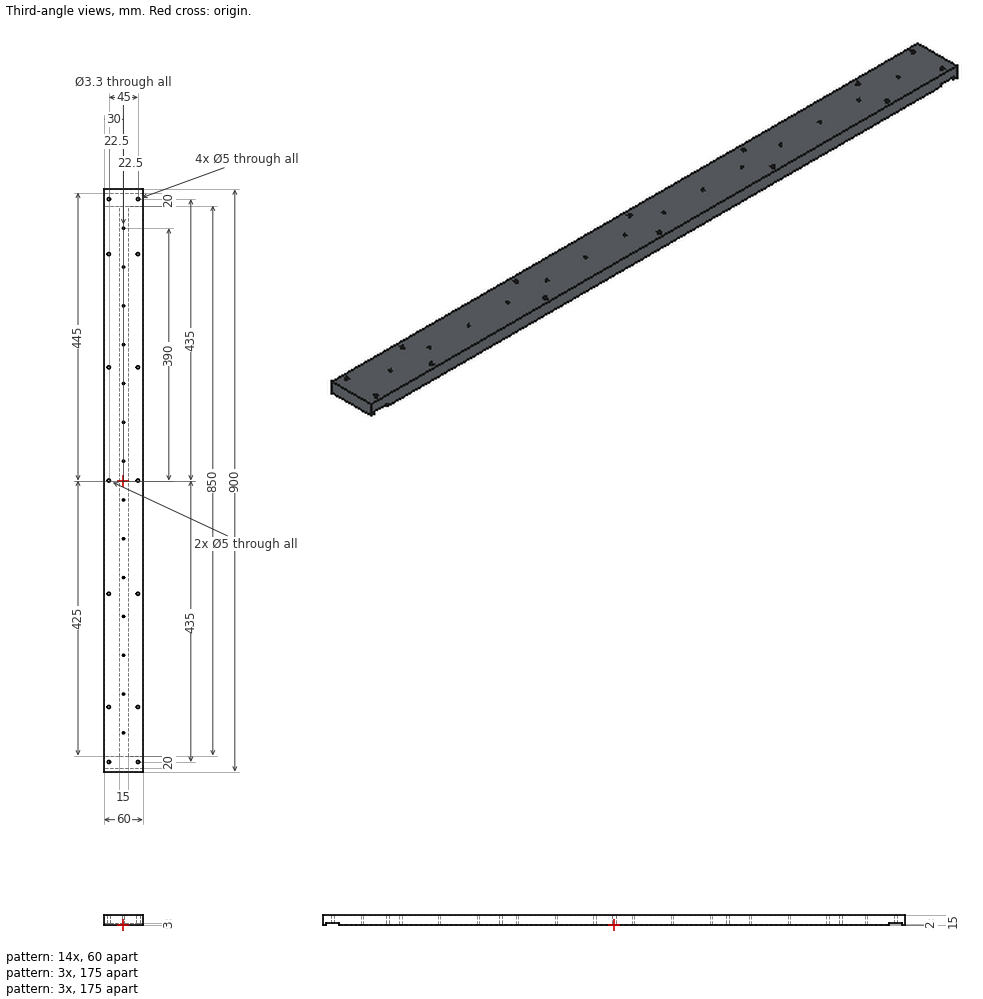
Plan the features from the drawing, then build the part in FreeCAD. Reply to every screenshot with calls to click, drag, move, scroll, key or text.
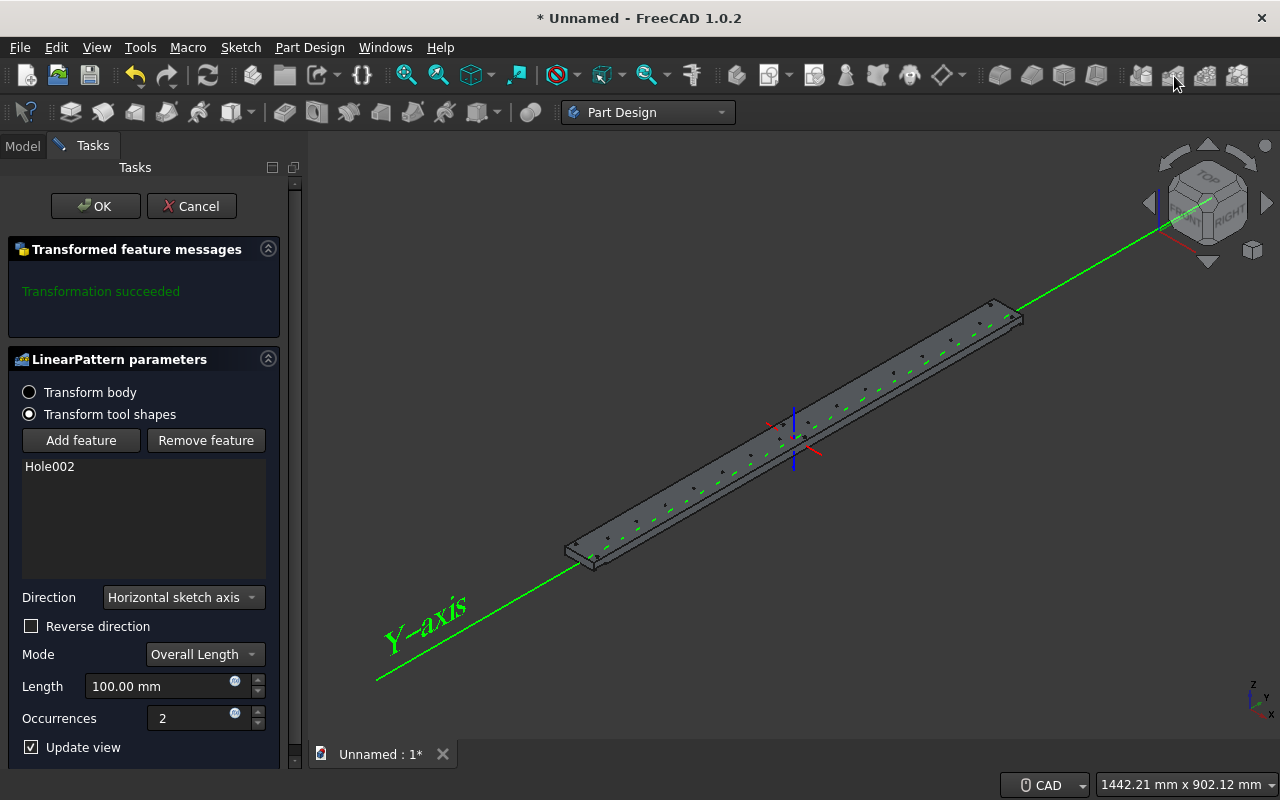
click(184, 598)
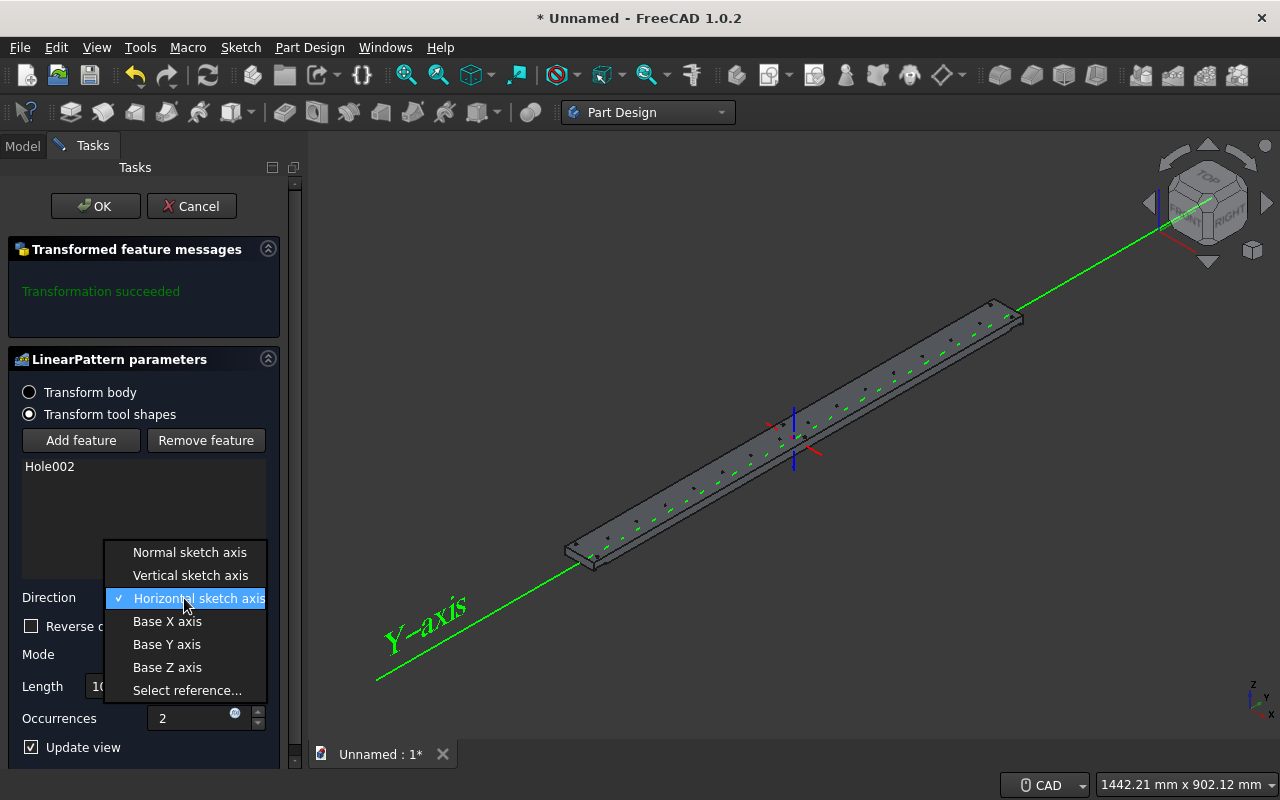
click(184, 644)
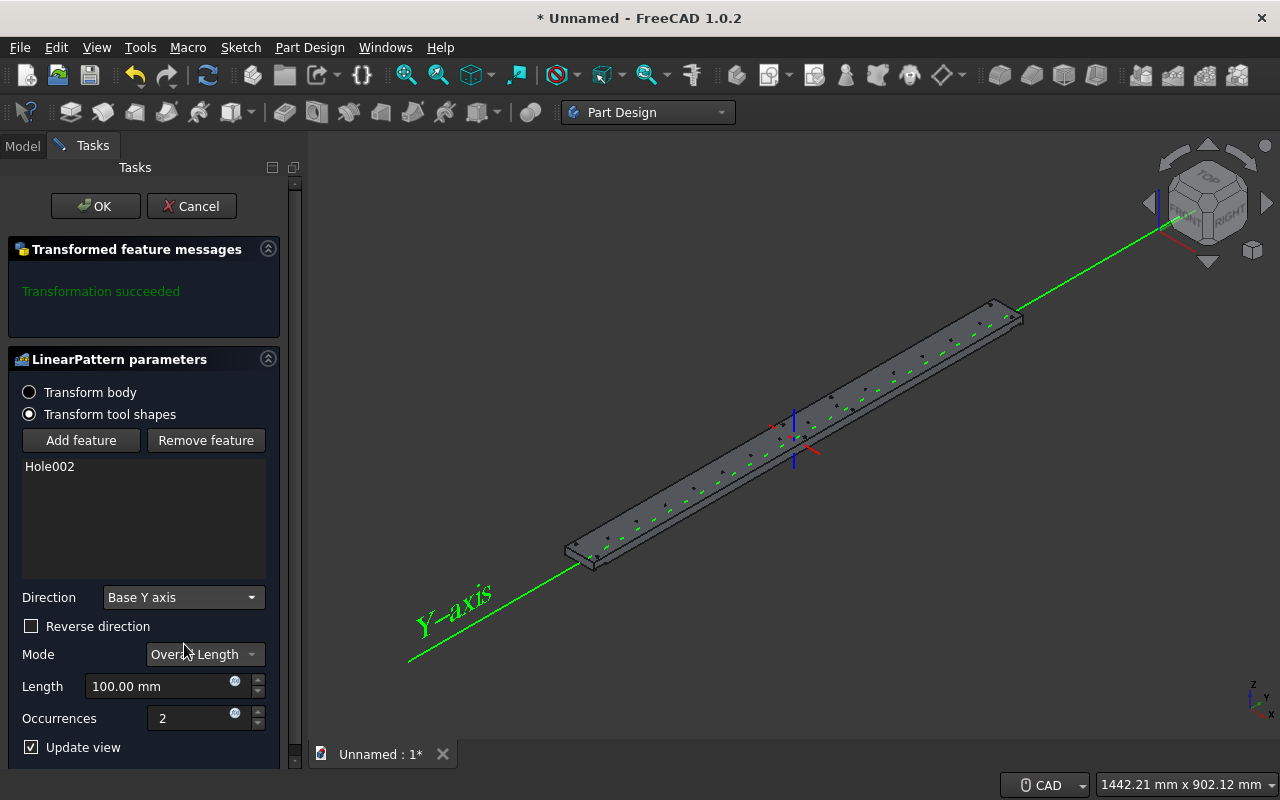
click(206, 654)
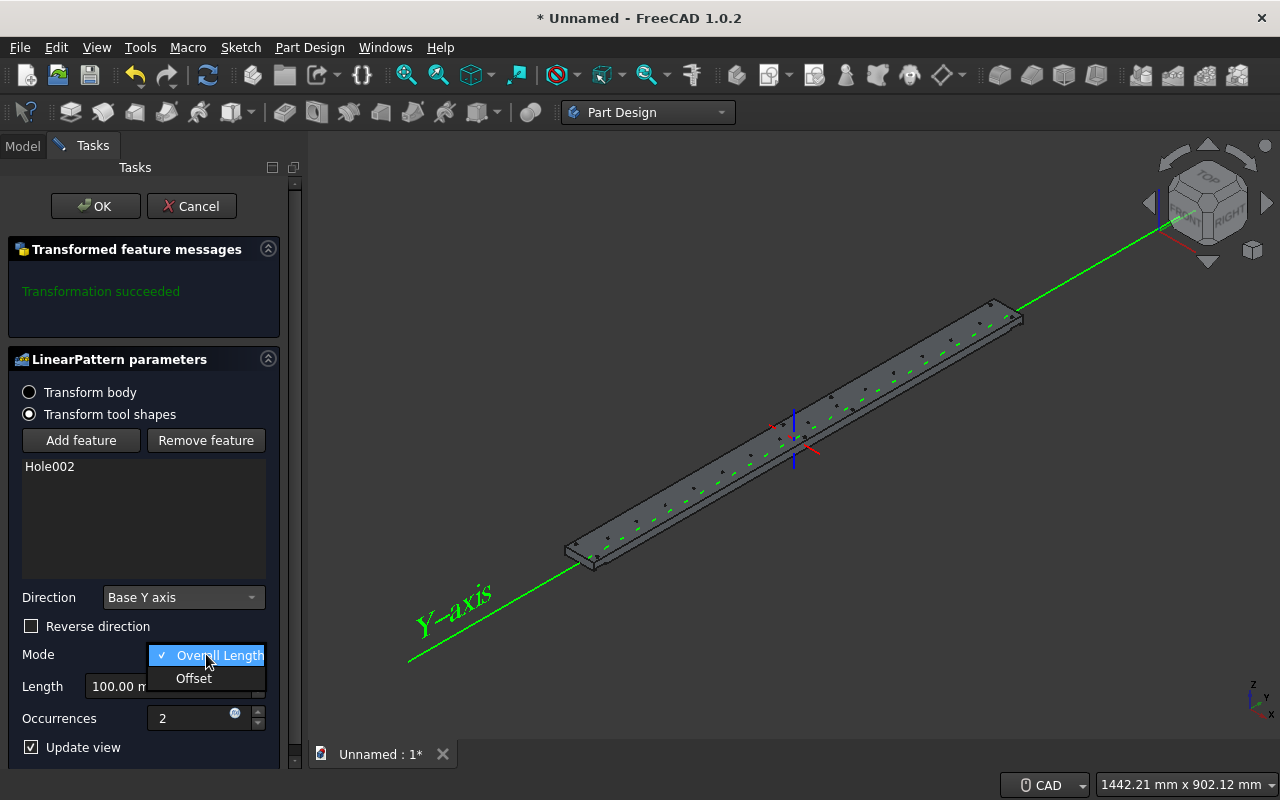
click(206, 678)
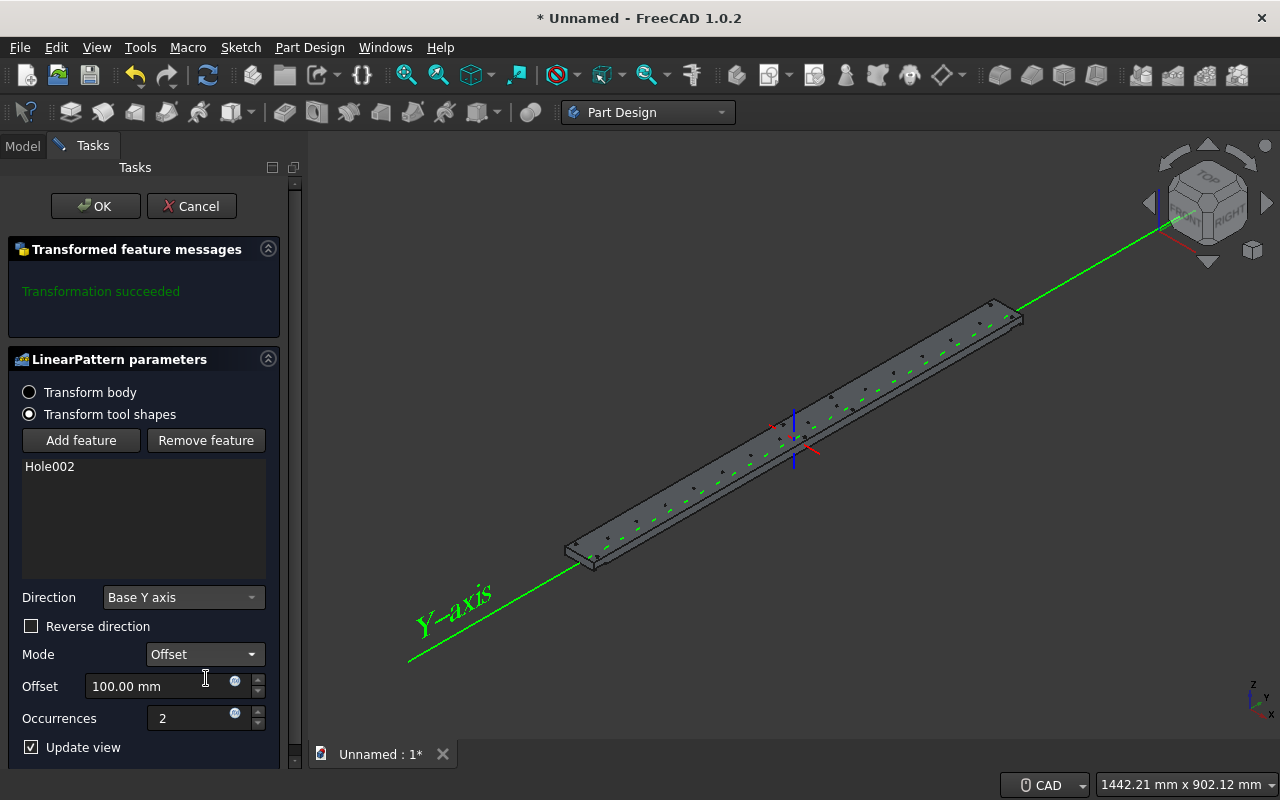
triple_click(168, 686)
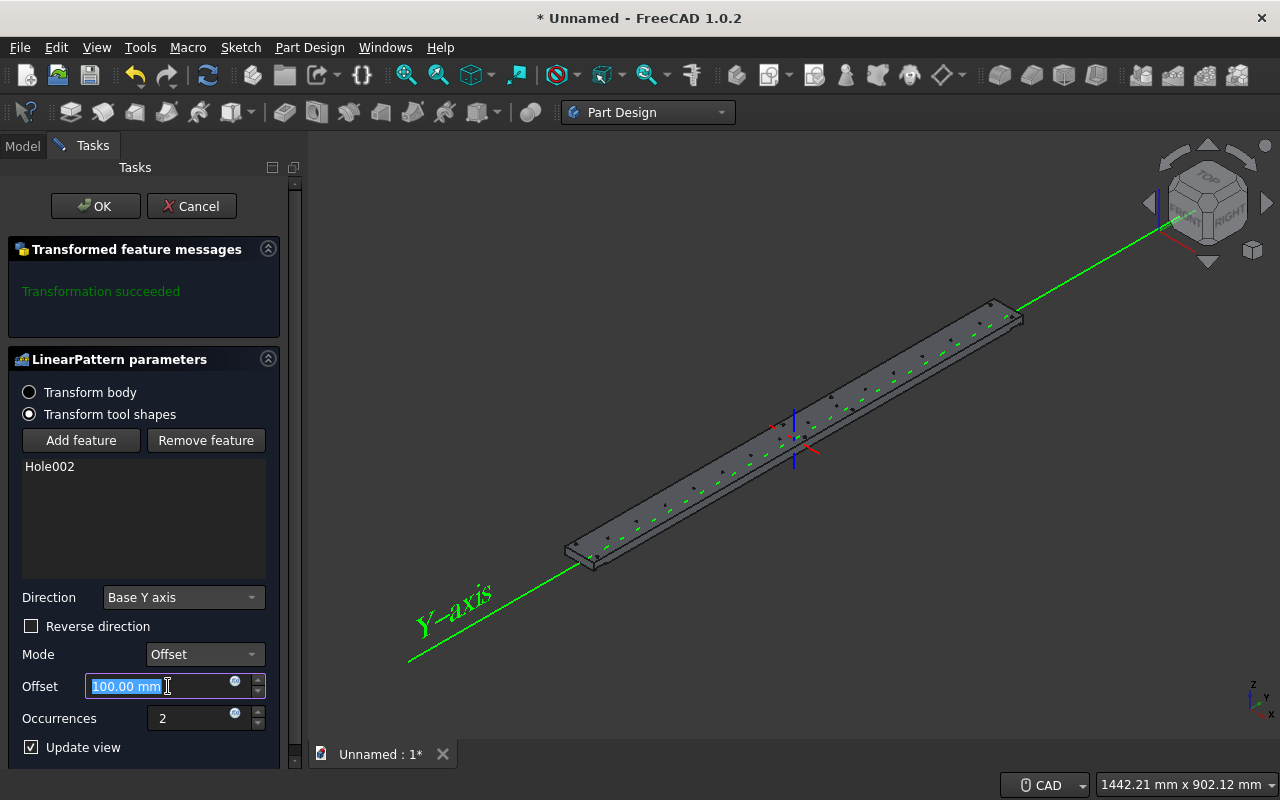
text(175)
key(Tab)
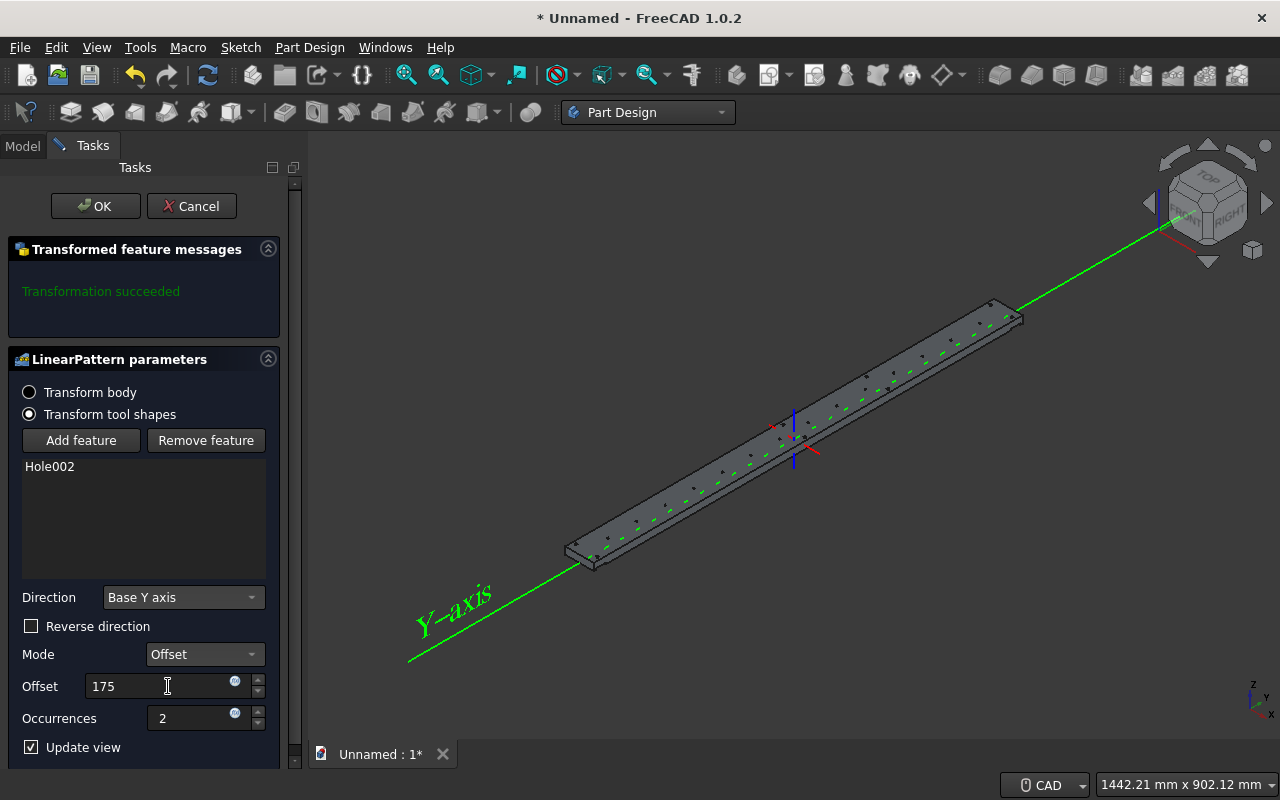
triple_click(198, 718)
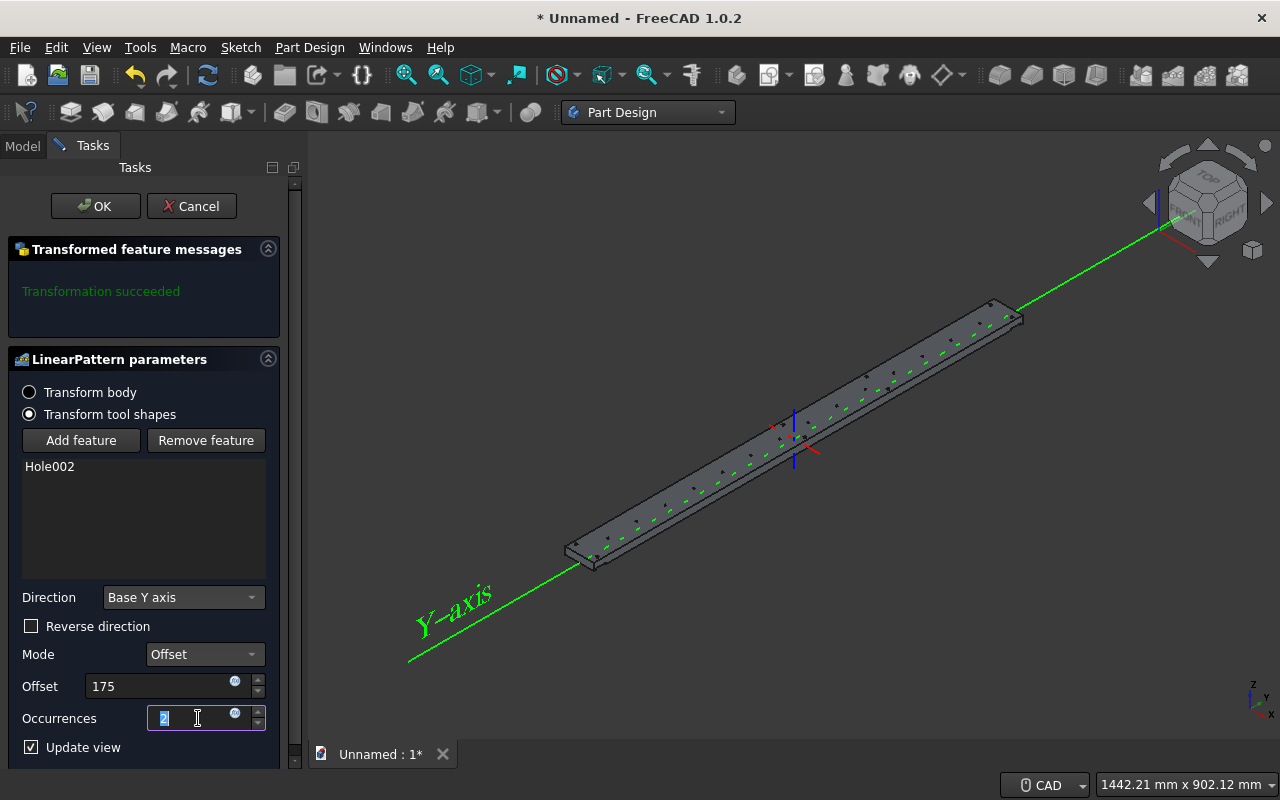
text(3)
key(Tab)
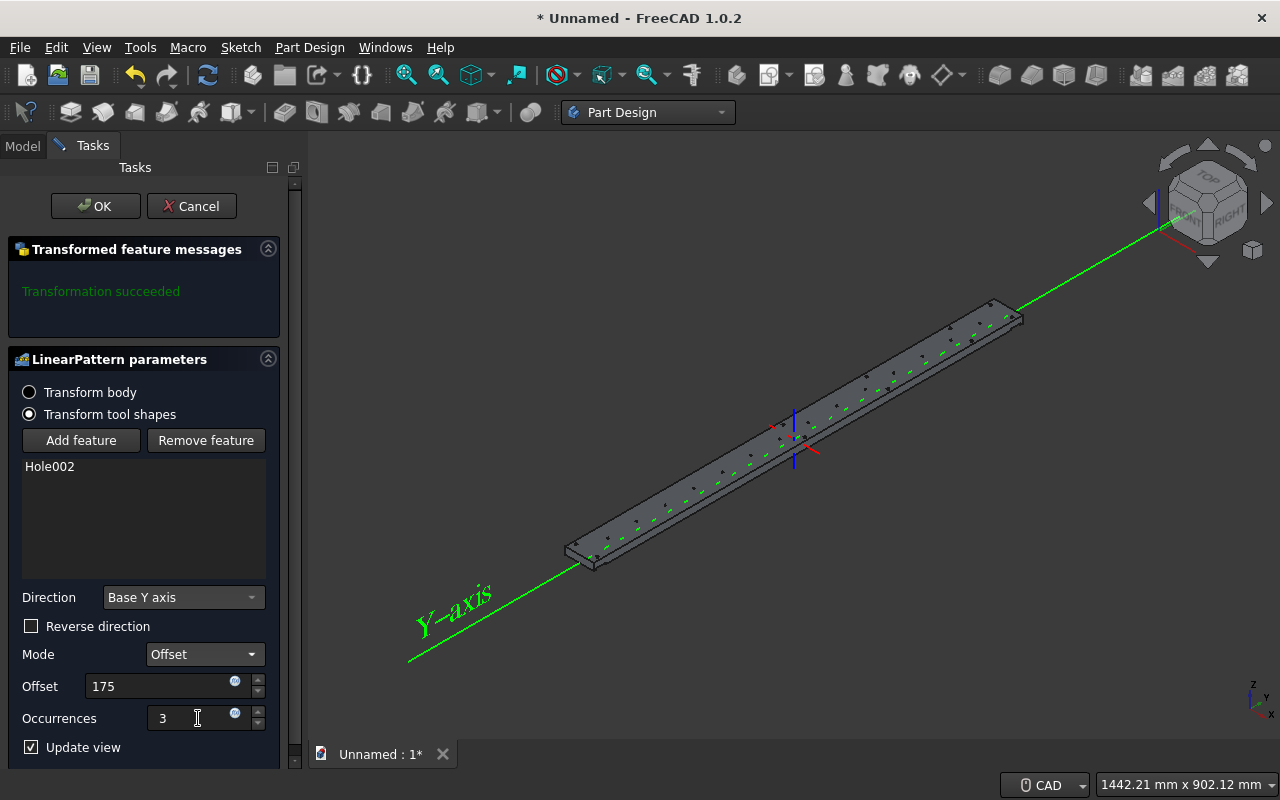
click(30, 626)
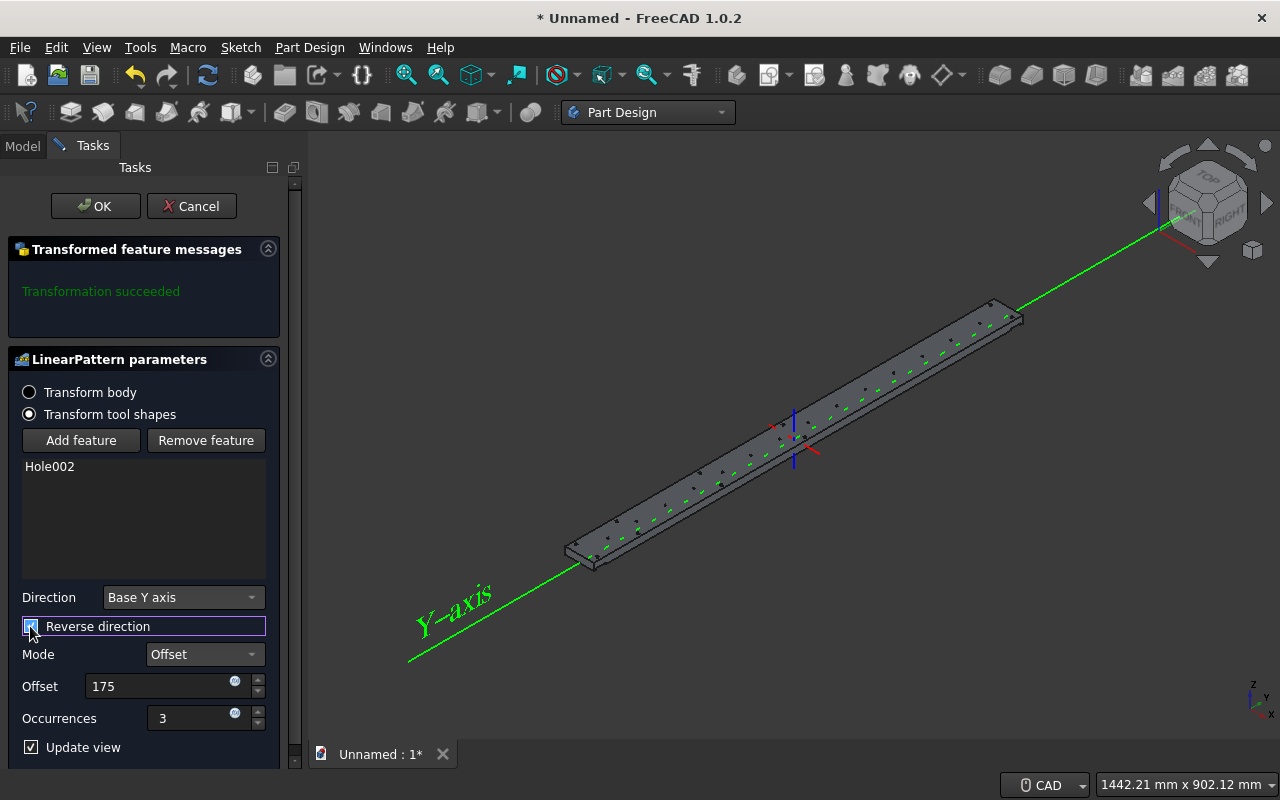
click(96, 206)